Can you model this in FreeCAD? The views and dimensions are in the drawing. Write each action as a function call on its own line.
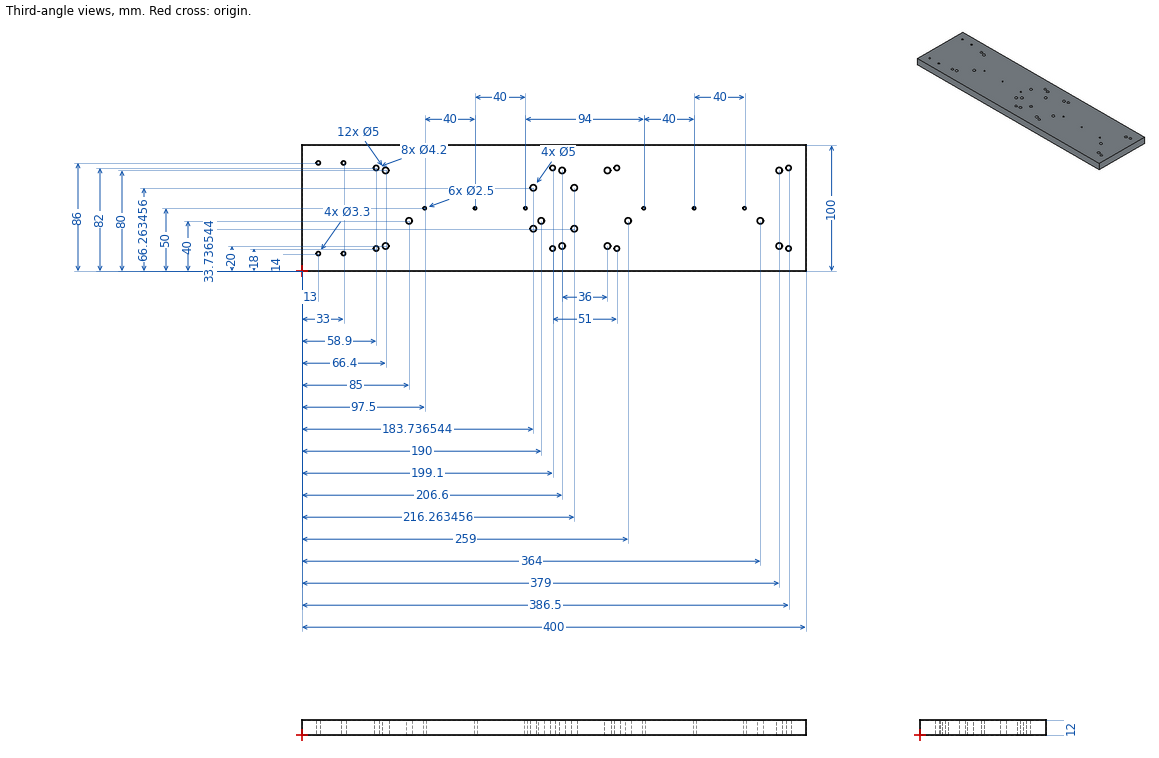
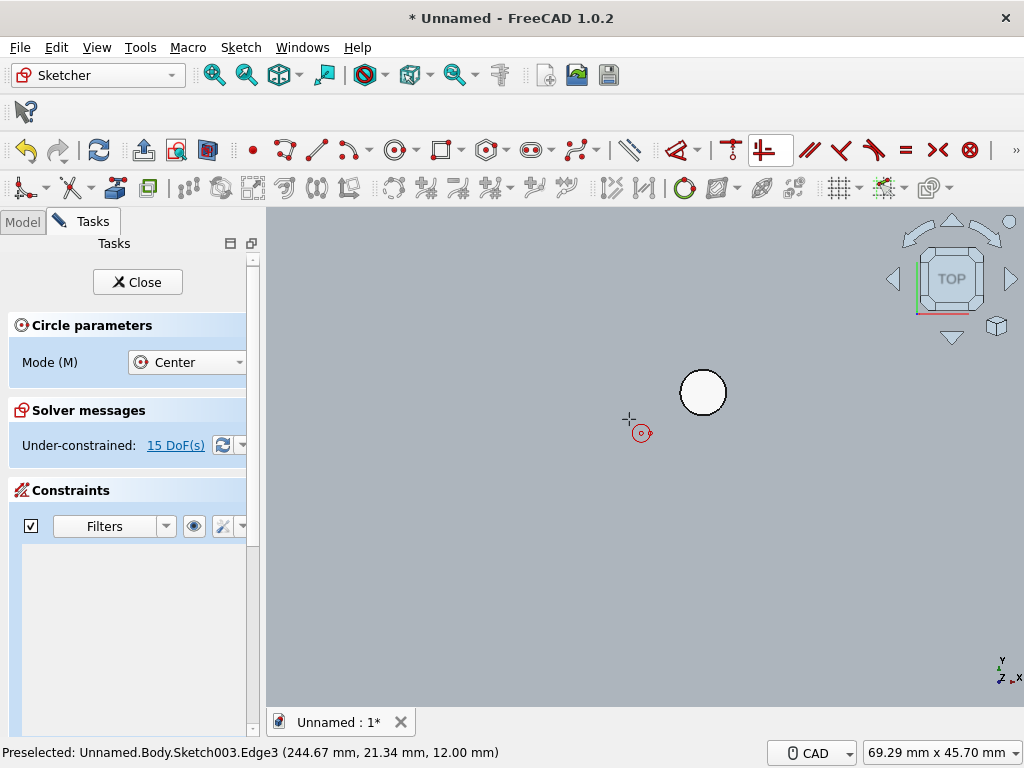
scroll(629, 419, down, 12)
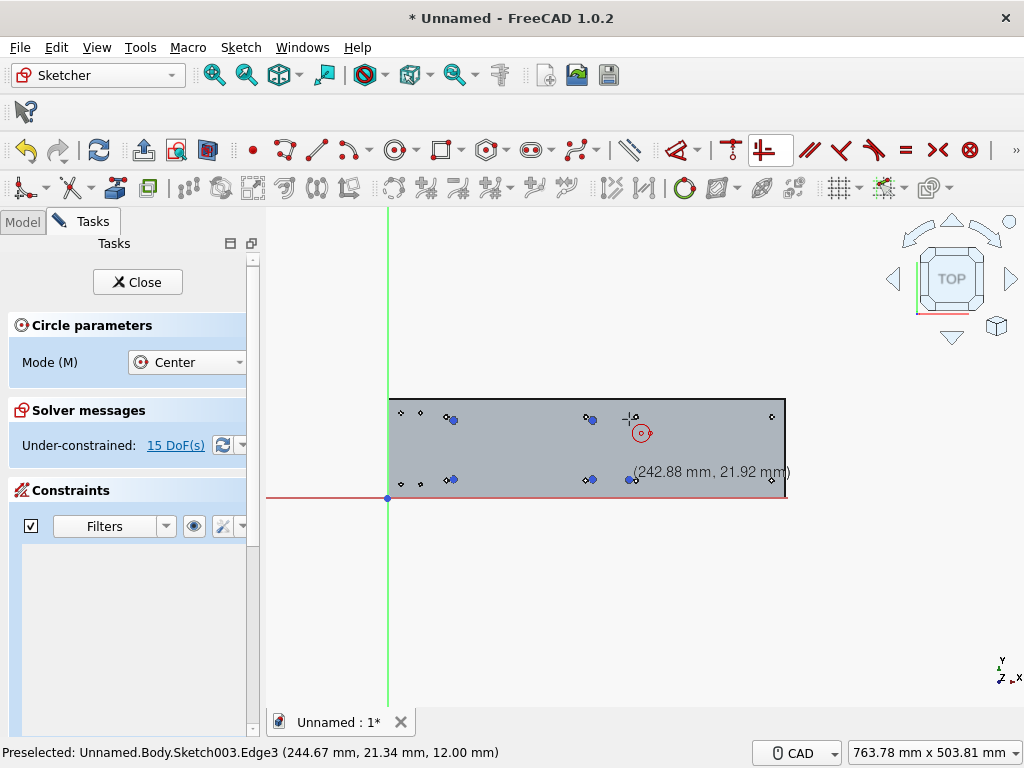
click(629, 419)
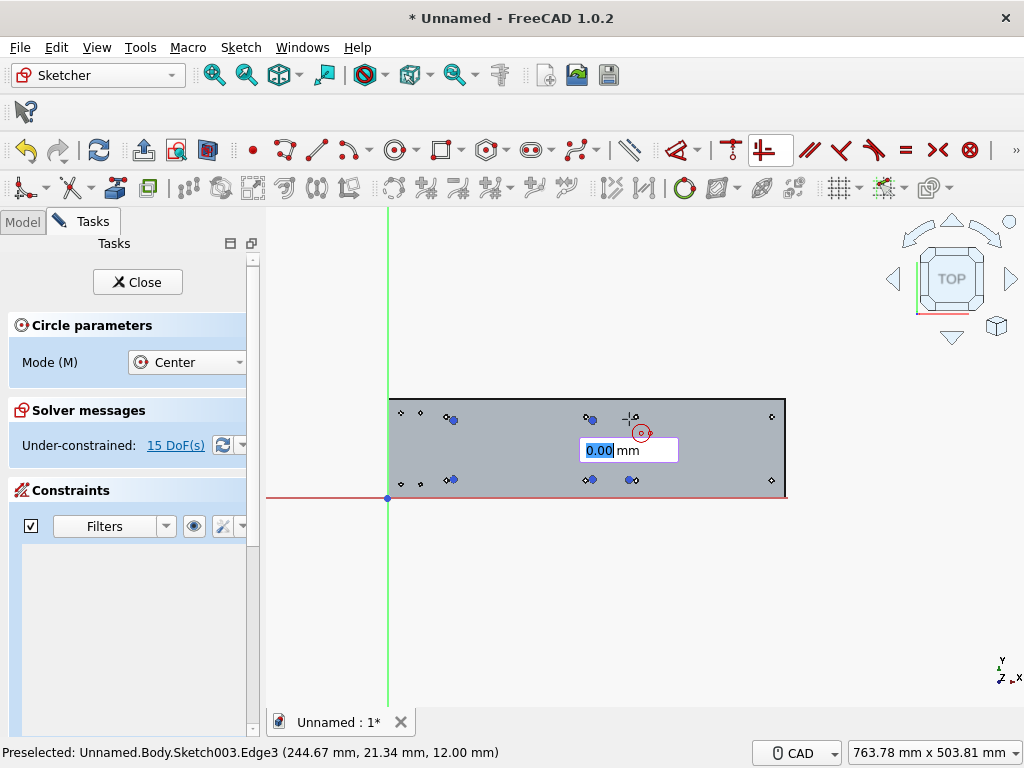
scroll(630, 417, up, 10)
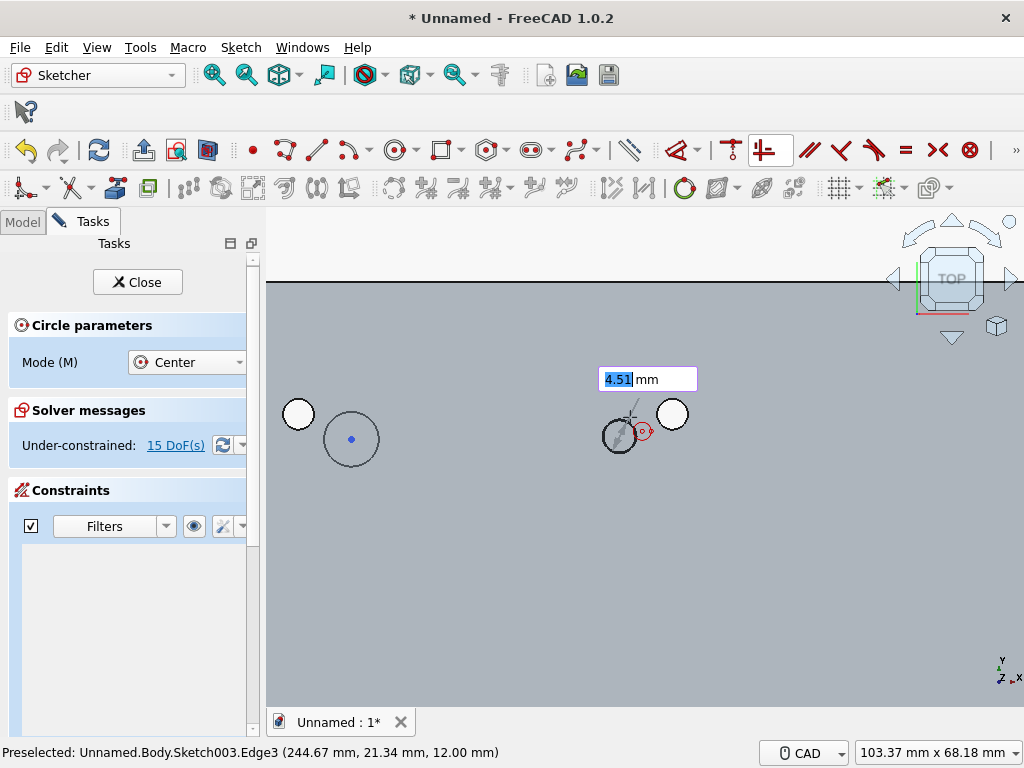
click(630, 416)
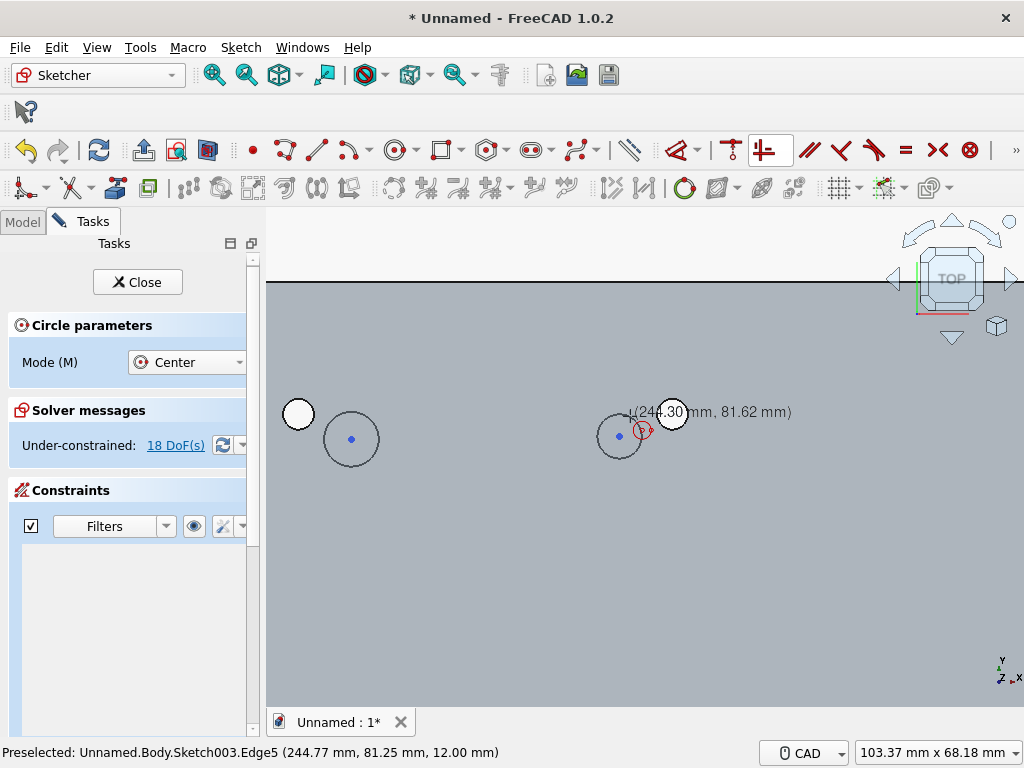
scroll(630, 417, down, 10)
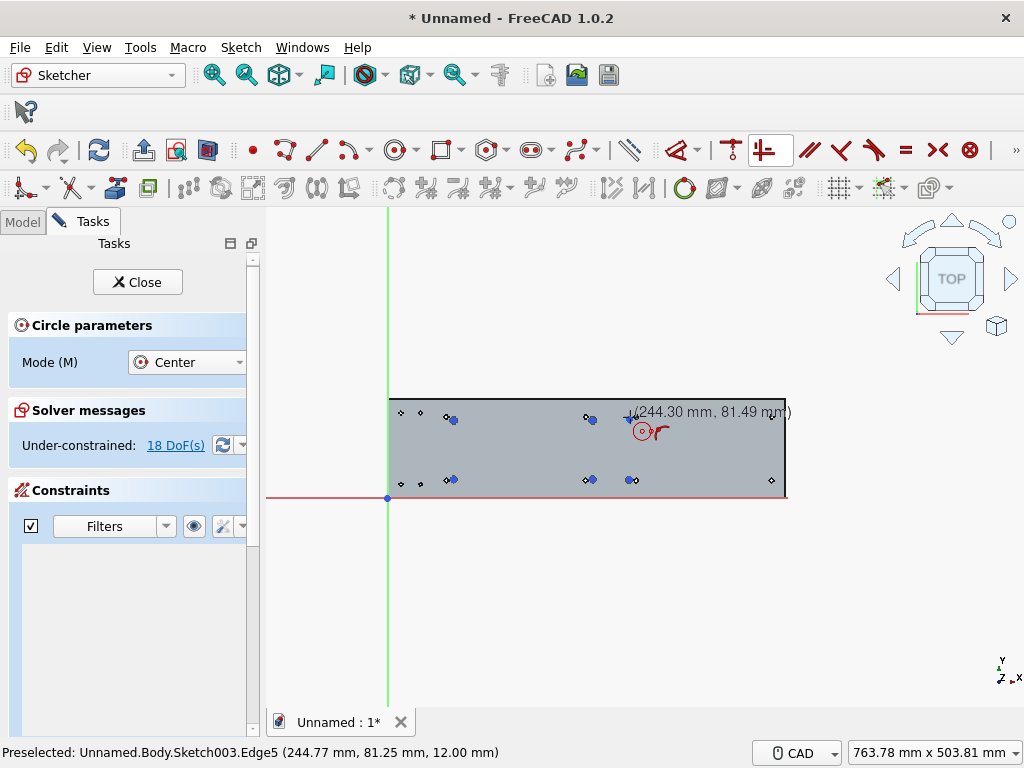
scroll(764, 419, up, 12)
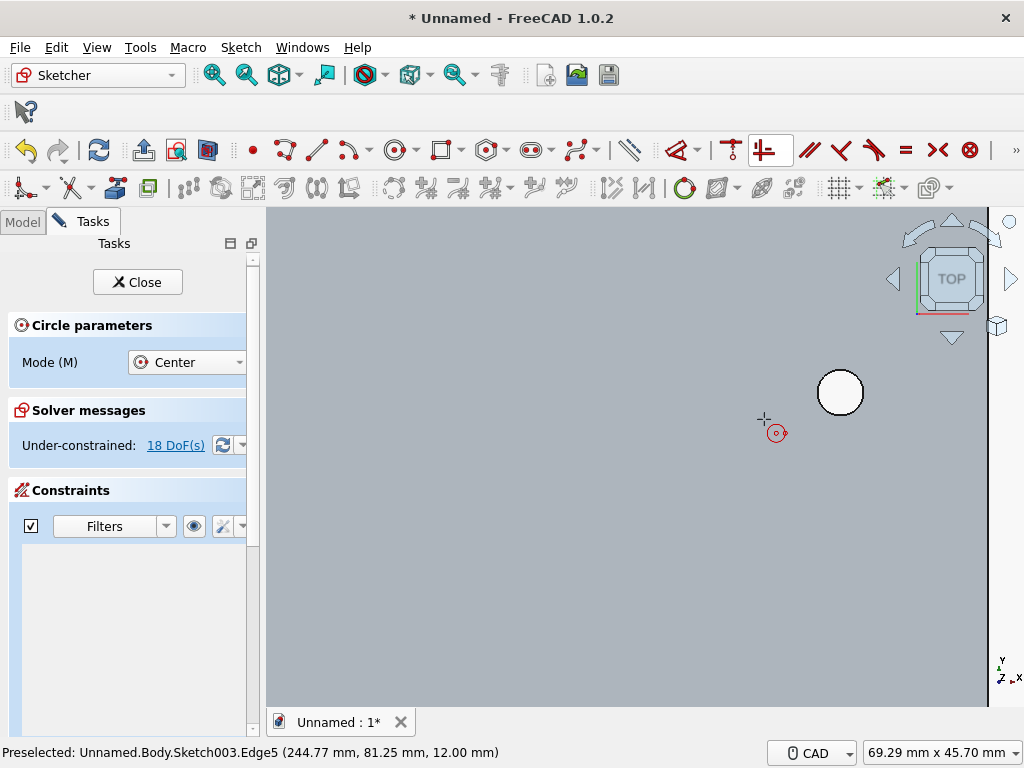
scroll(764, 419, down, 12)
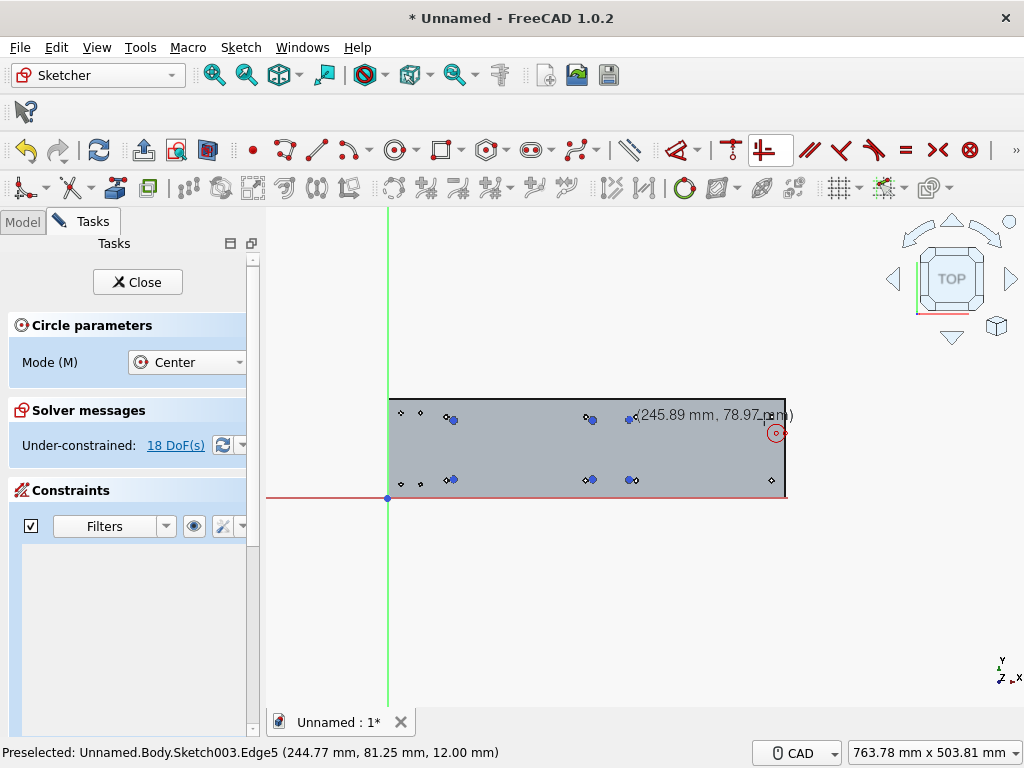
click(764, 419)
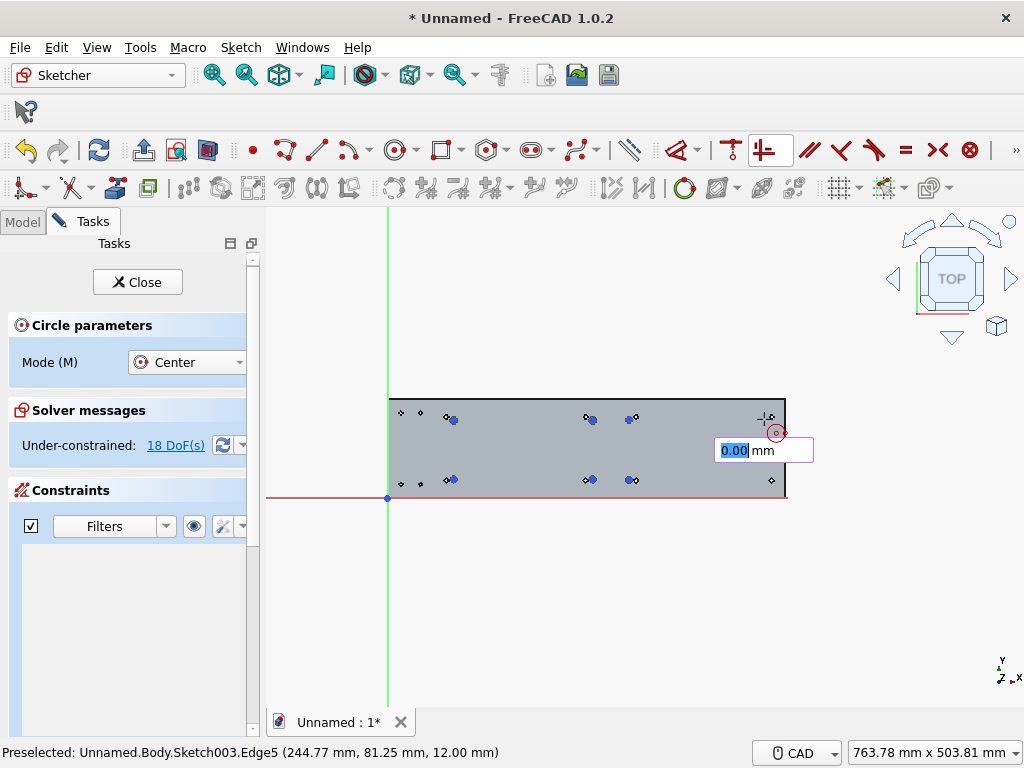
scroll(766, 417, up, 10)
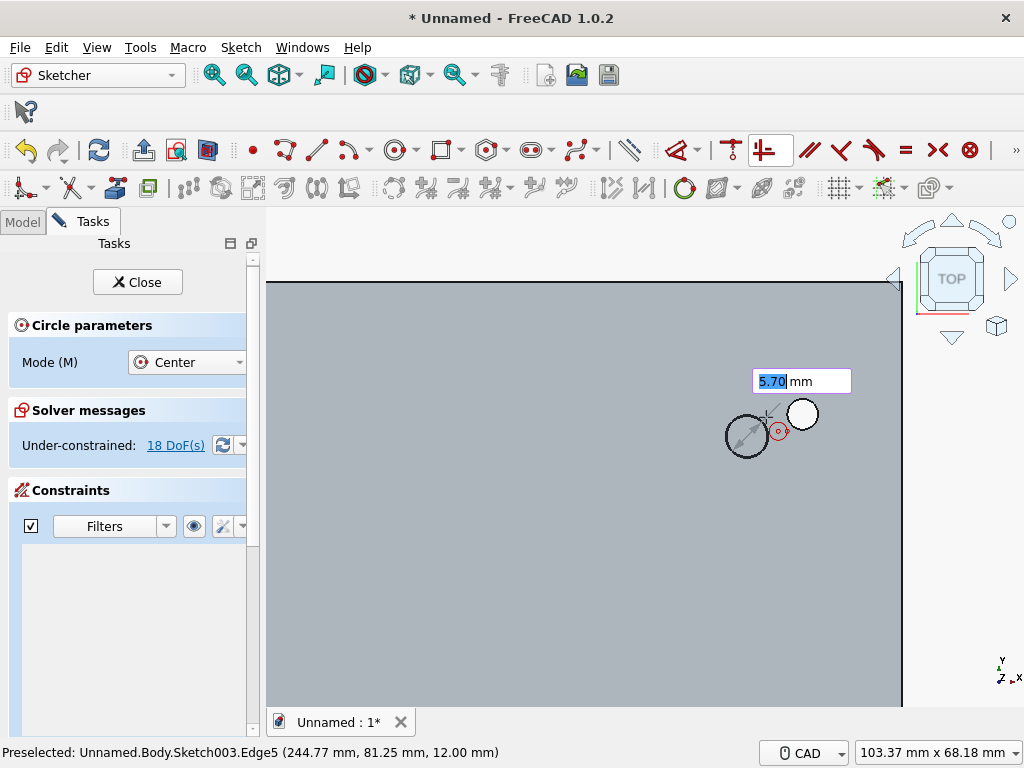
click(761, 416)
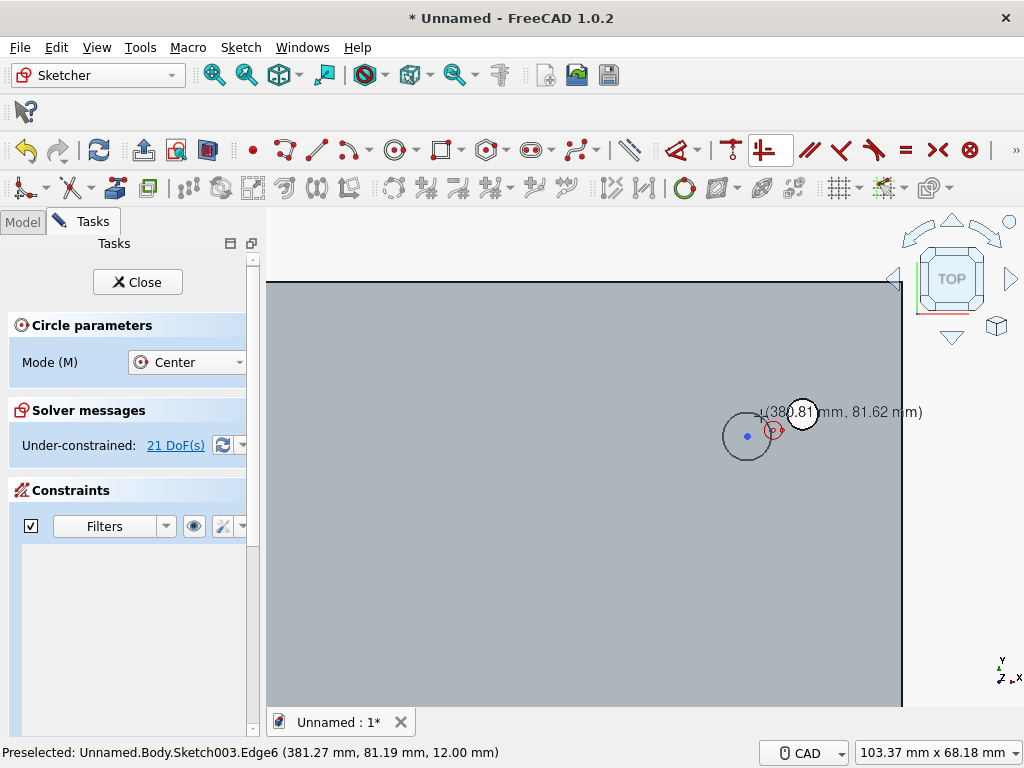
scroll(766, 417, down, 10)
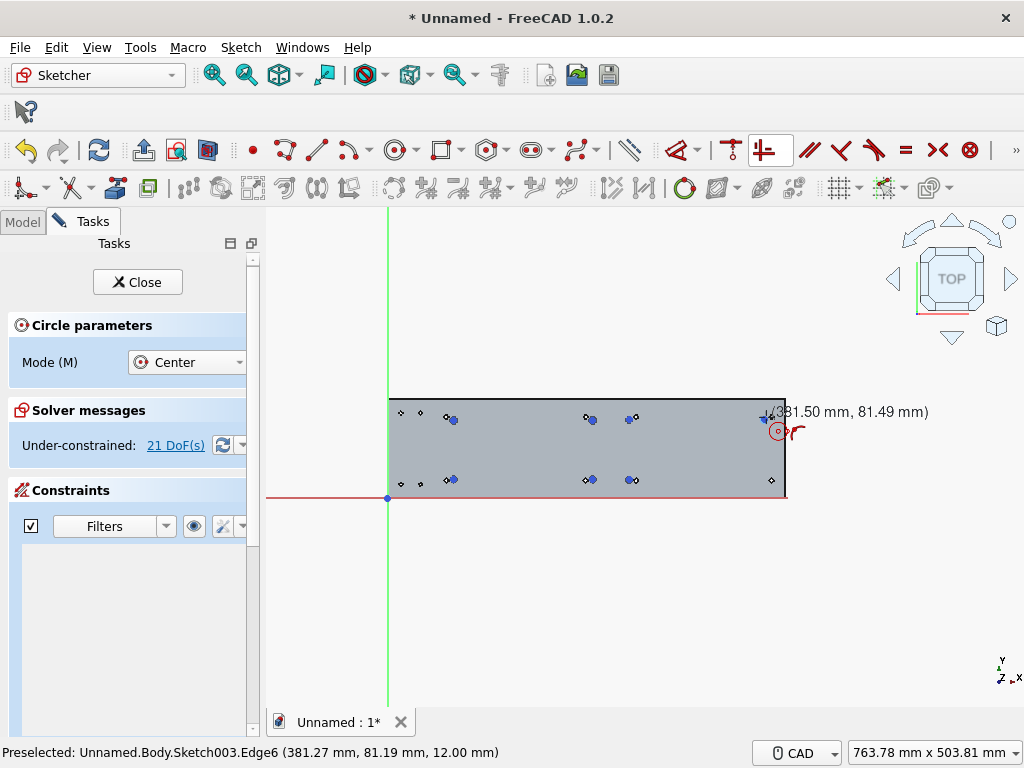
scroll(764, 479, up, 12)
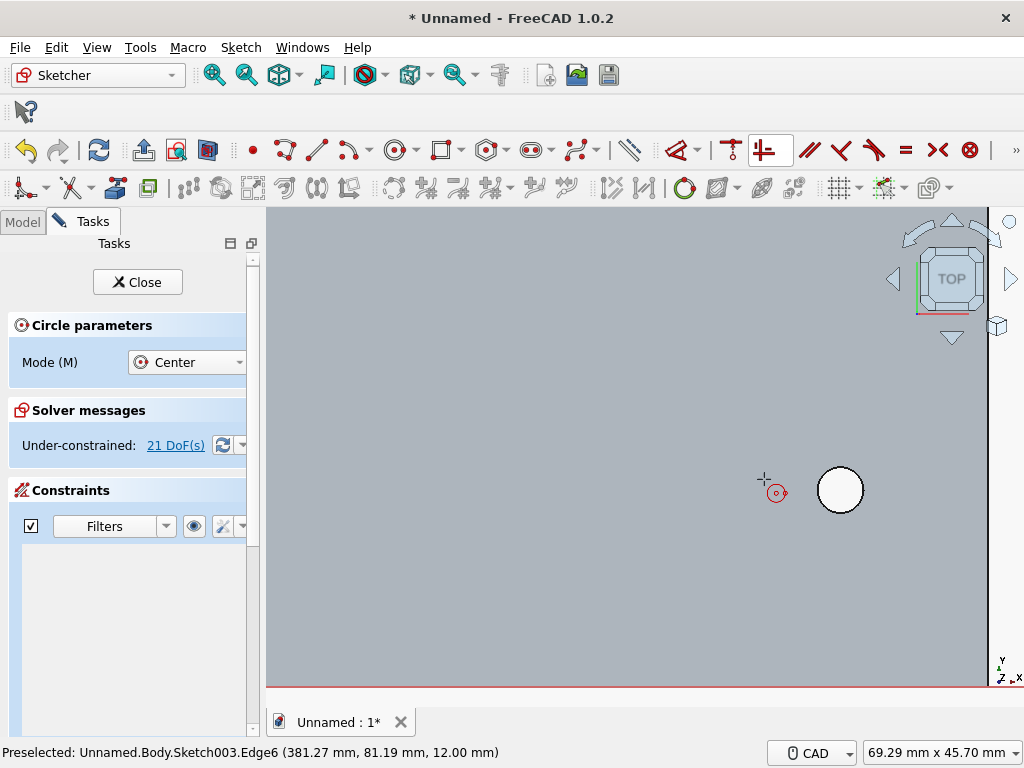
scroll(764, 479, down, 12)